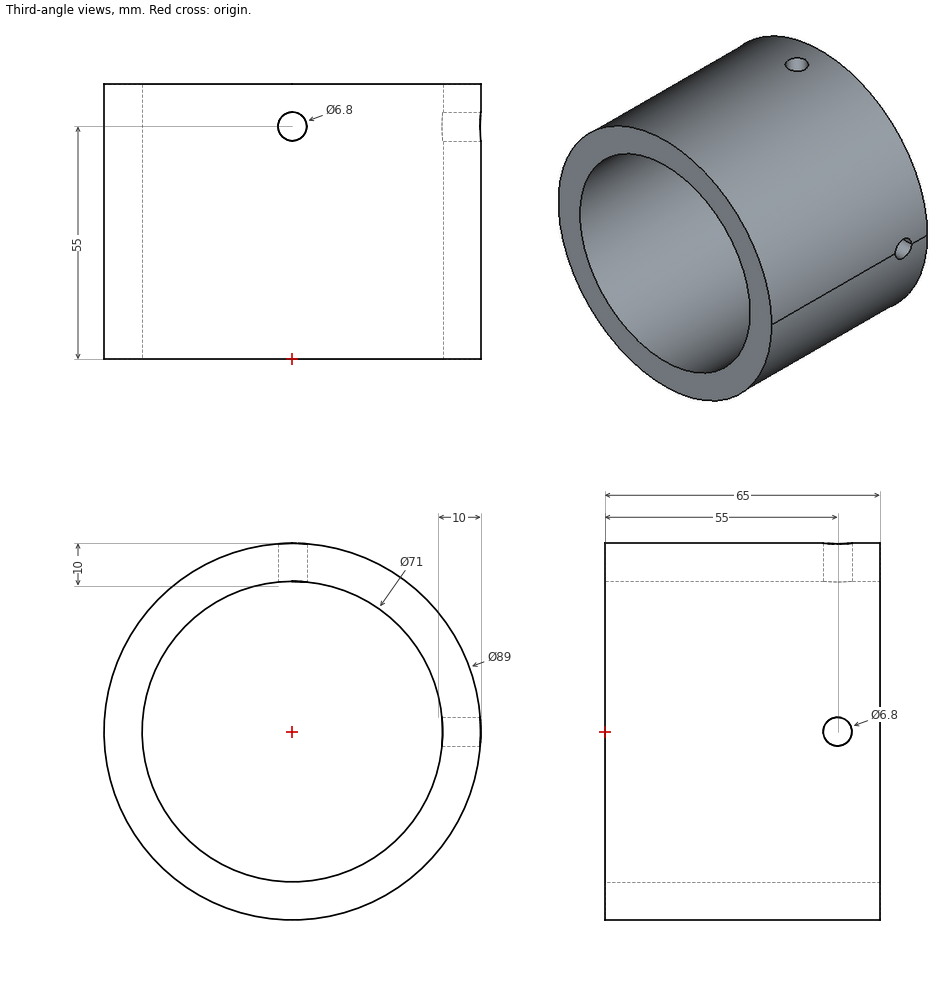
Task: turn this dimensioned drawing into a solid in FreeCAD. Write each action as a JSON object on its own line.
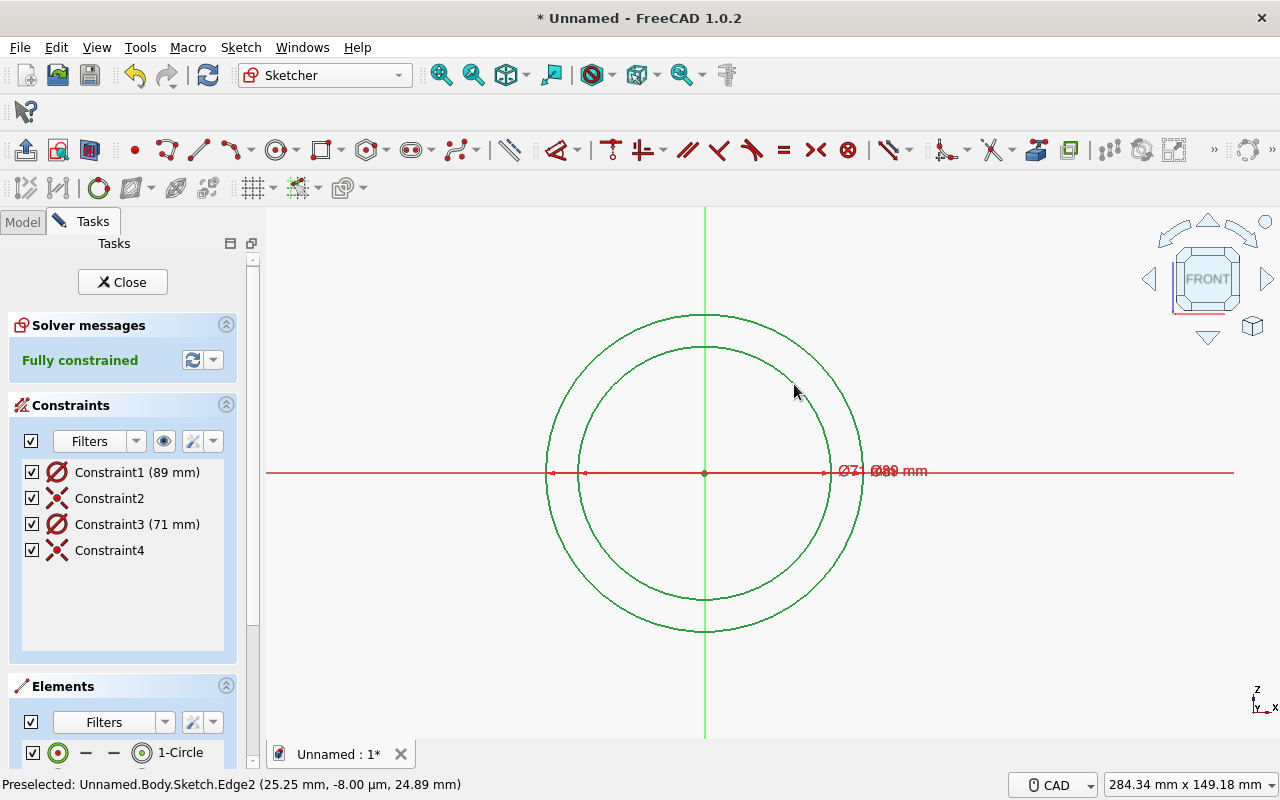
{"action": "left_click", "coordinate": [123, 282]}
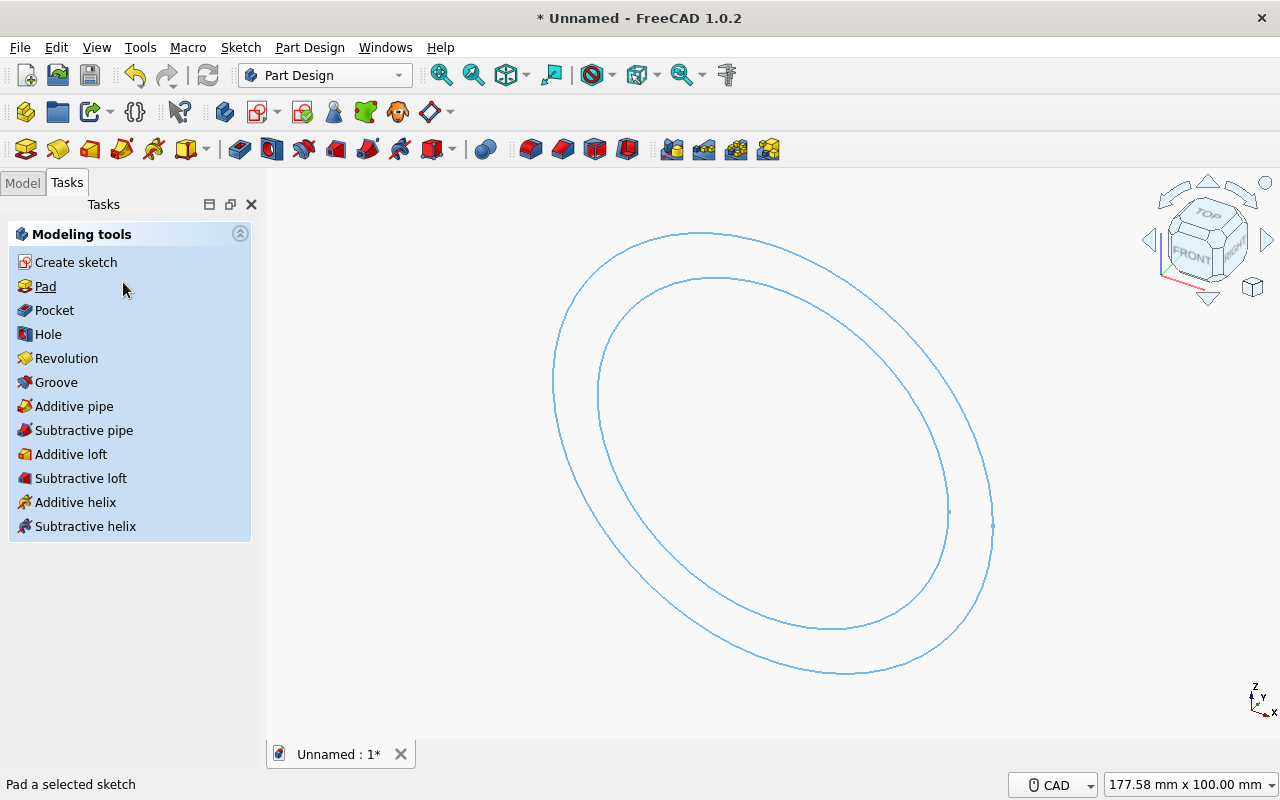
{"action": "left_click", "coordinate": [26, 150]}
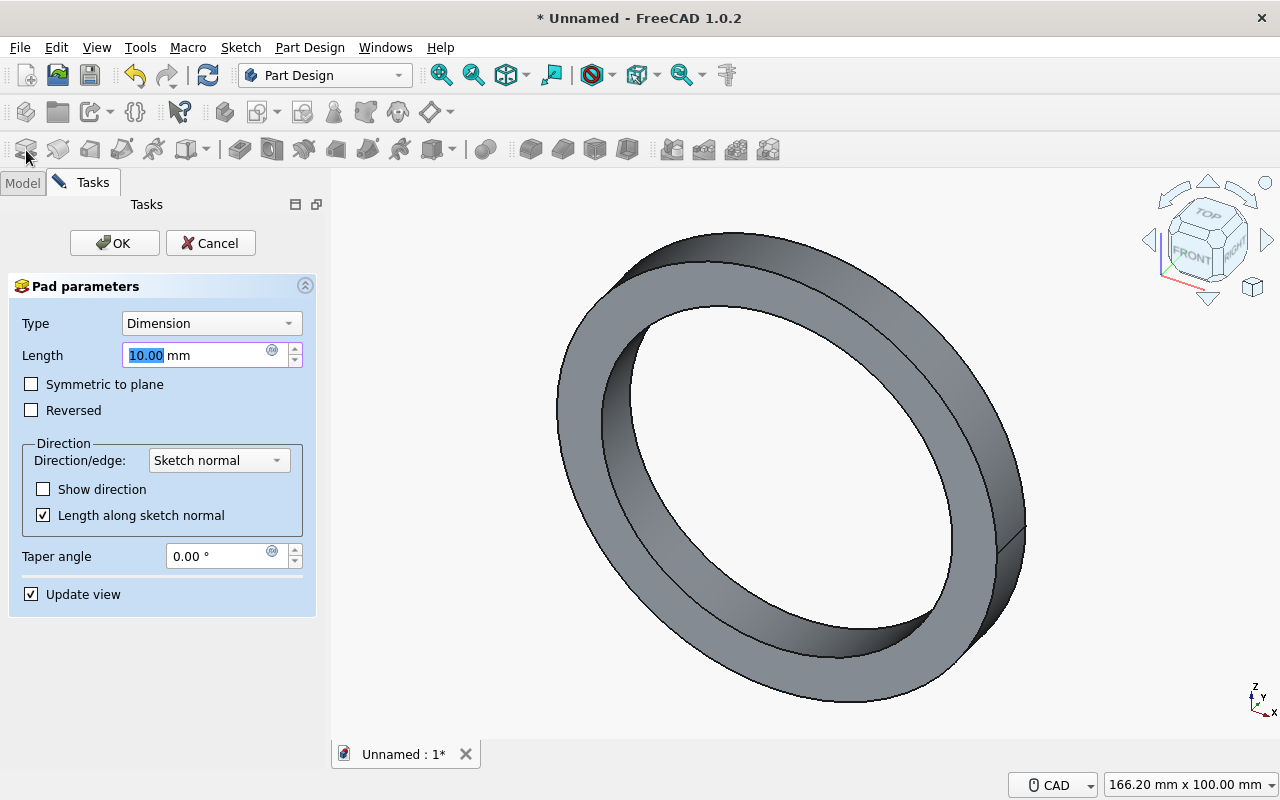
{"action": "type", "text": "65"}
{"action": "key", "text": "Tab"}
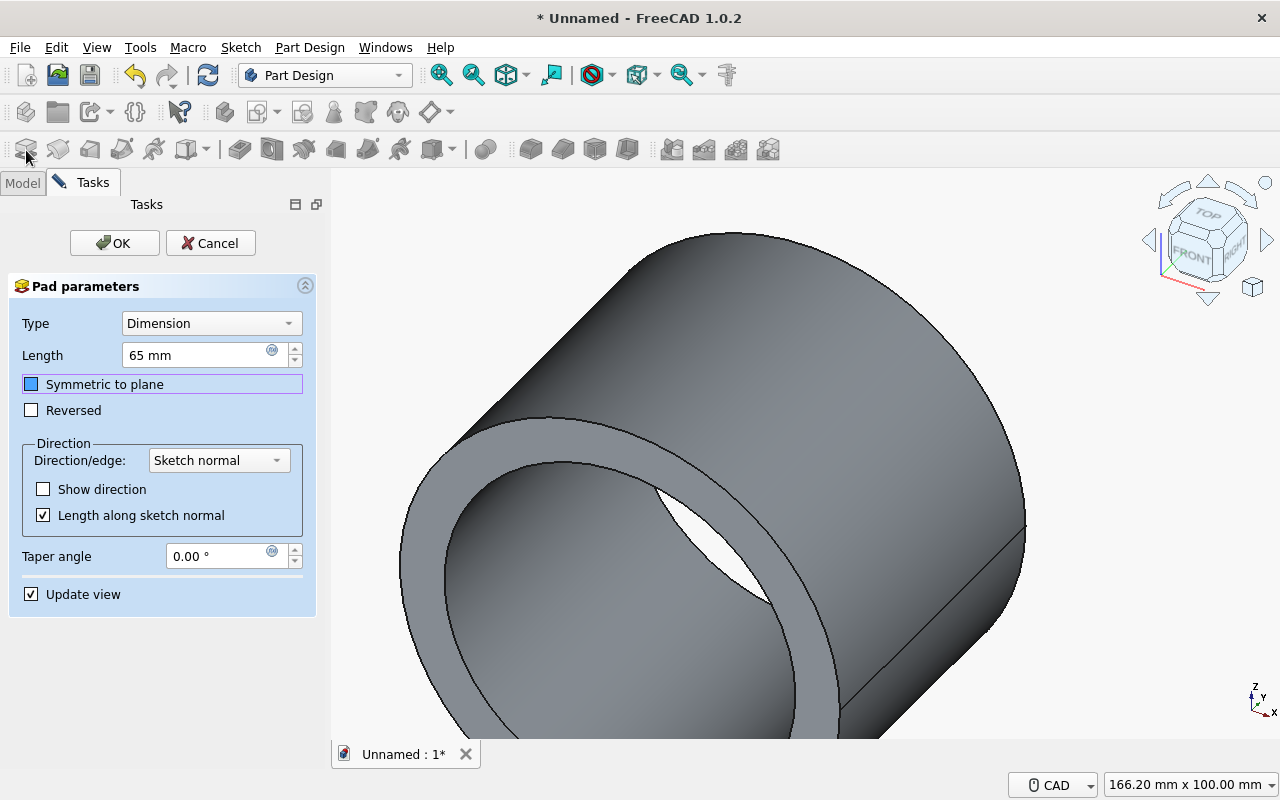
{"action": "left_click", "coordinate": [30, 410]}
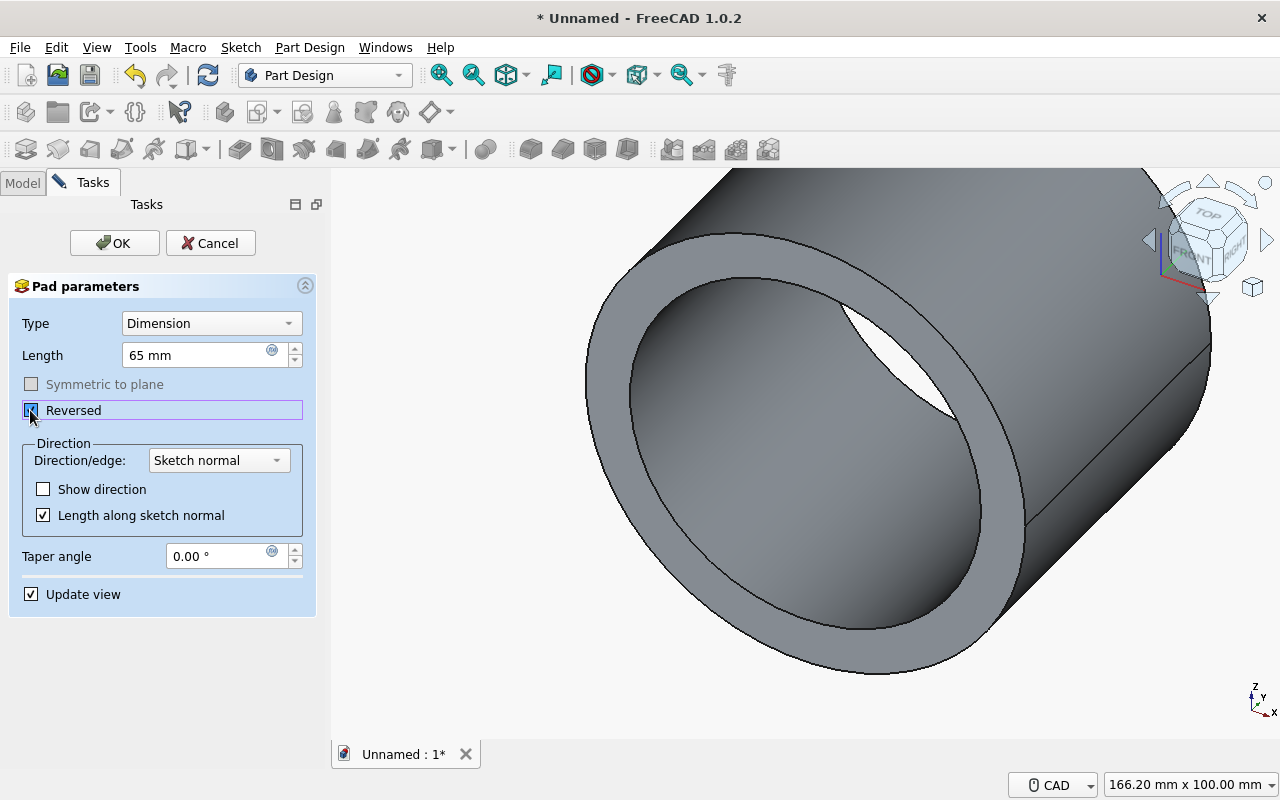
{"action": "left_click", "coordinate": [115, 243]}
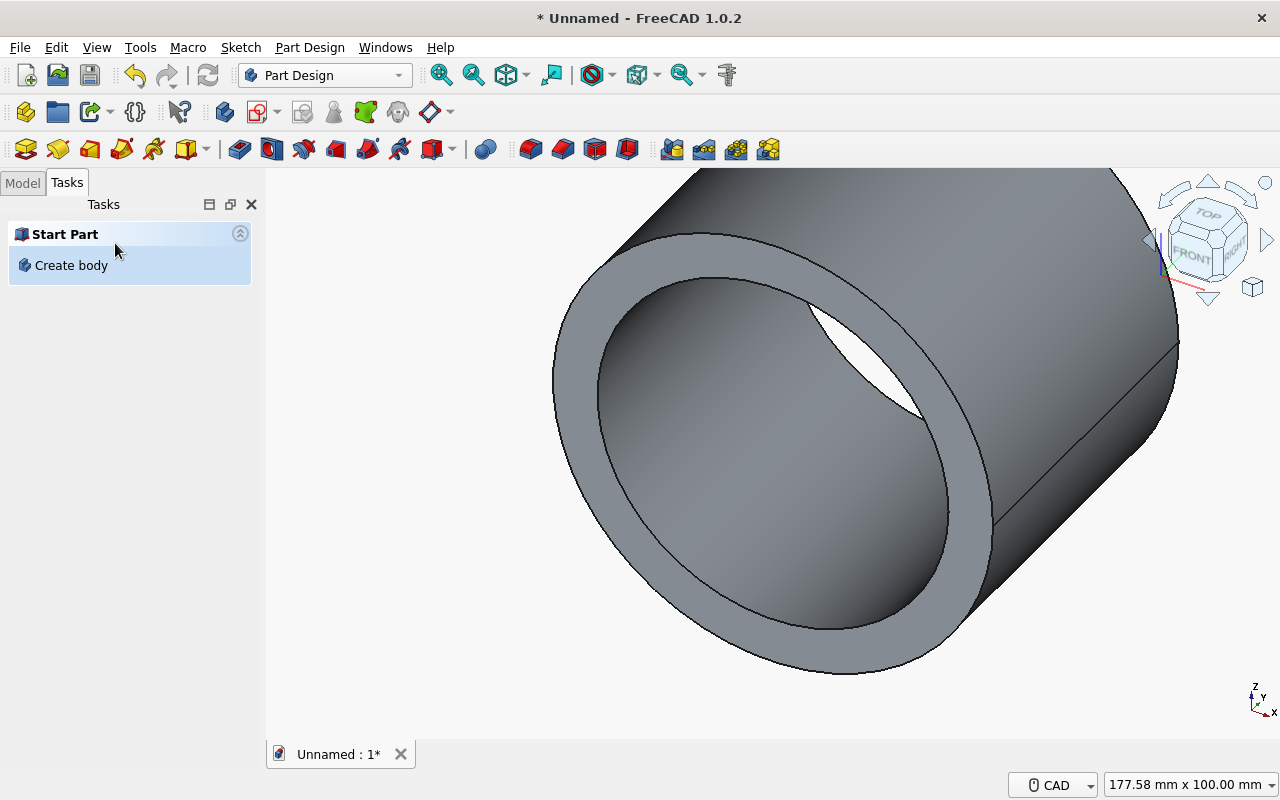
{"action": "key", "text": "v f"}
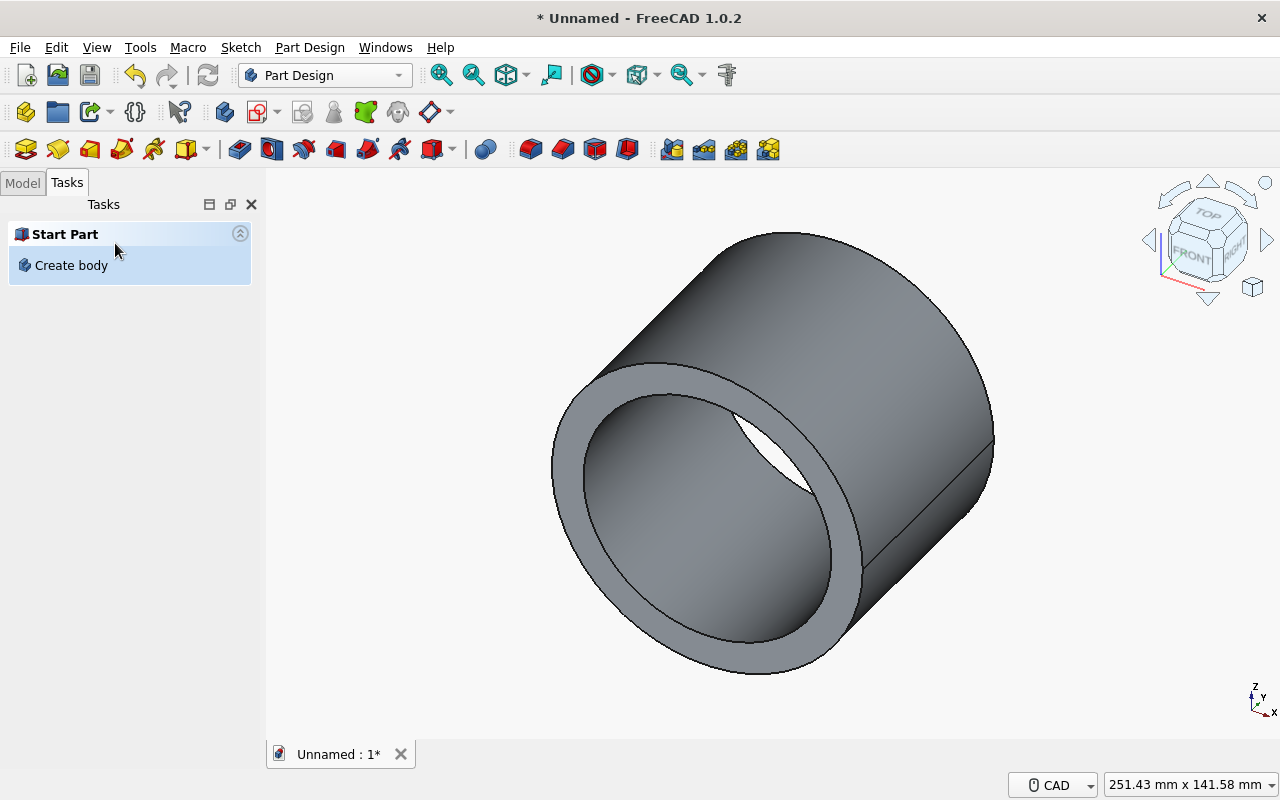
{"action": "left_click", "coordinate": [23, 182]}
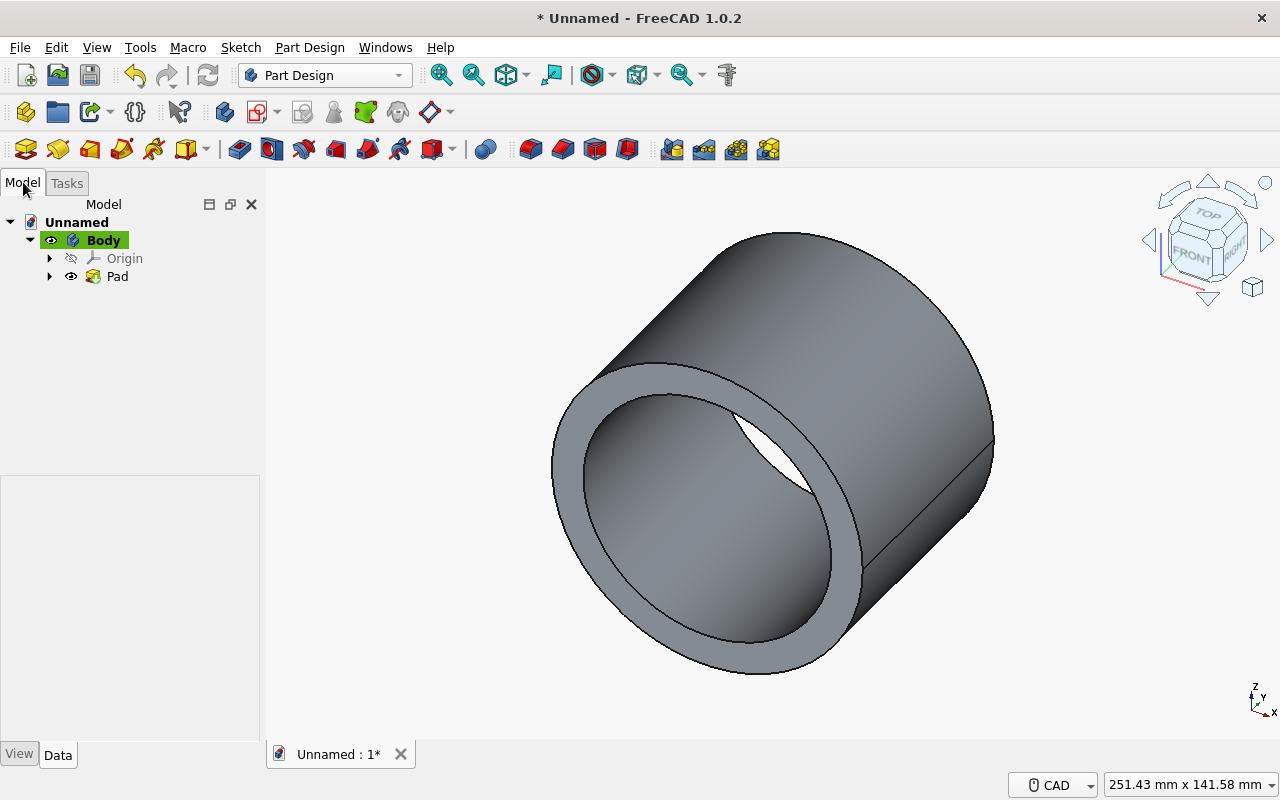
{"action": "left_click", "coordinate": [50, 258]}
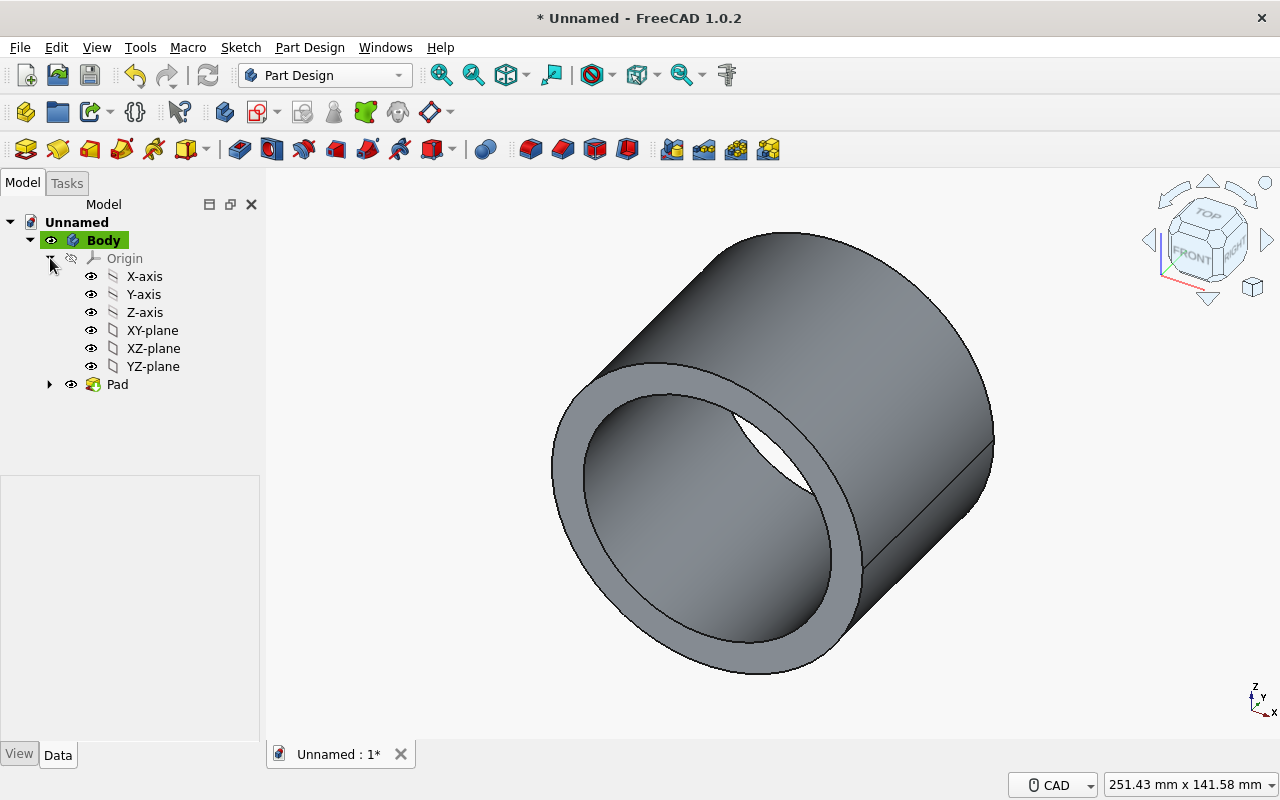
{"action": "left_click", "coordinate": [136, 366]}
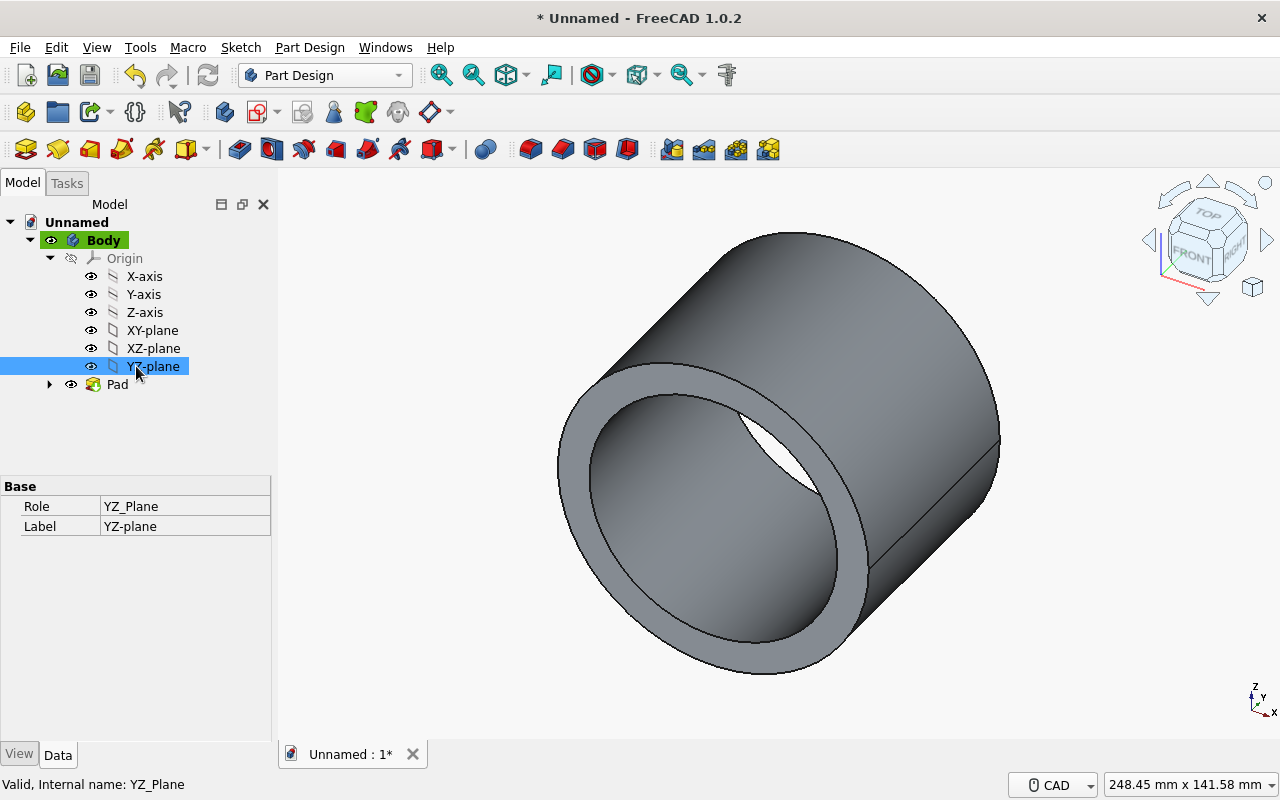
{"action": "left_click", "coordinate": [430, 112]}